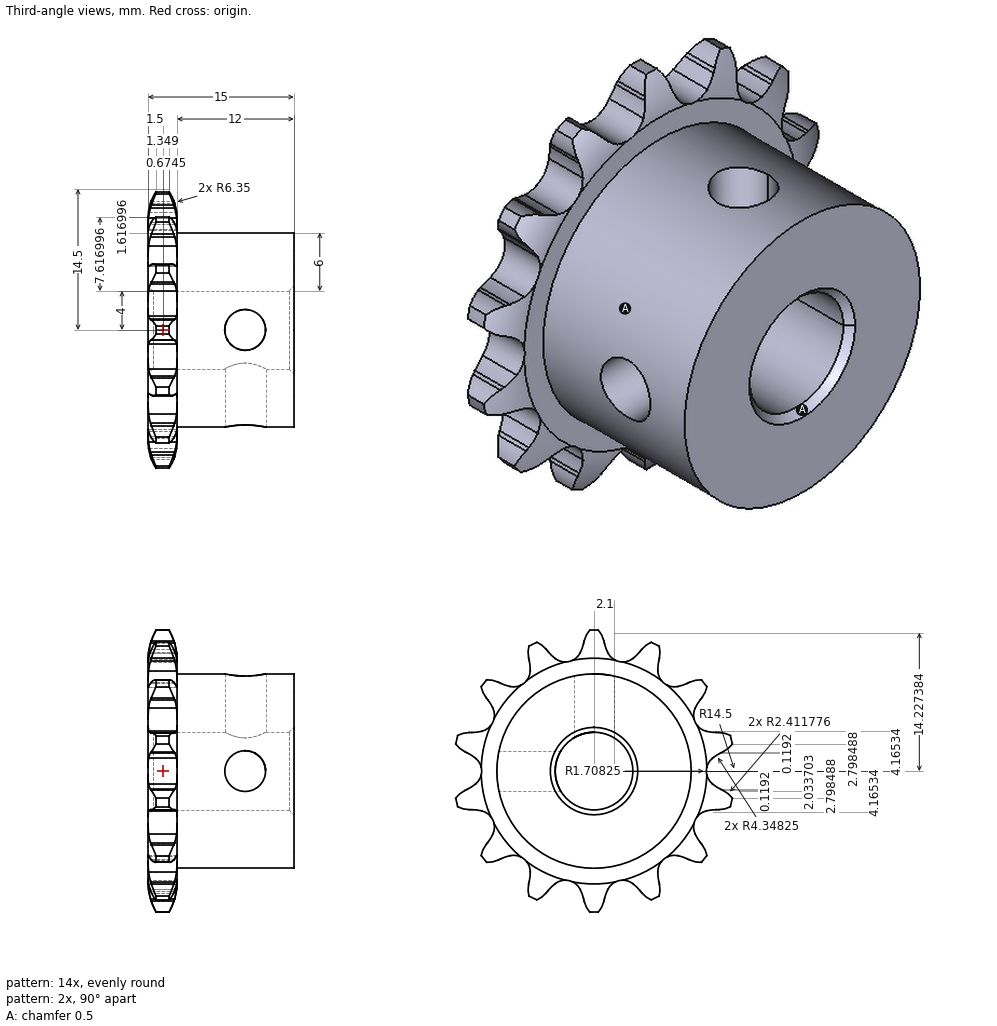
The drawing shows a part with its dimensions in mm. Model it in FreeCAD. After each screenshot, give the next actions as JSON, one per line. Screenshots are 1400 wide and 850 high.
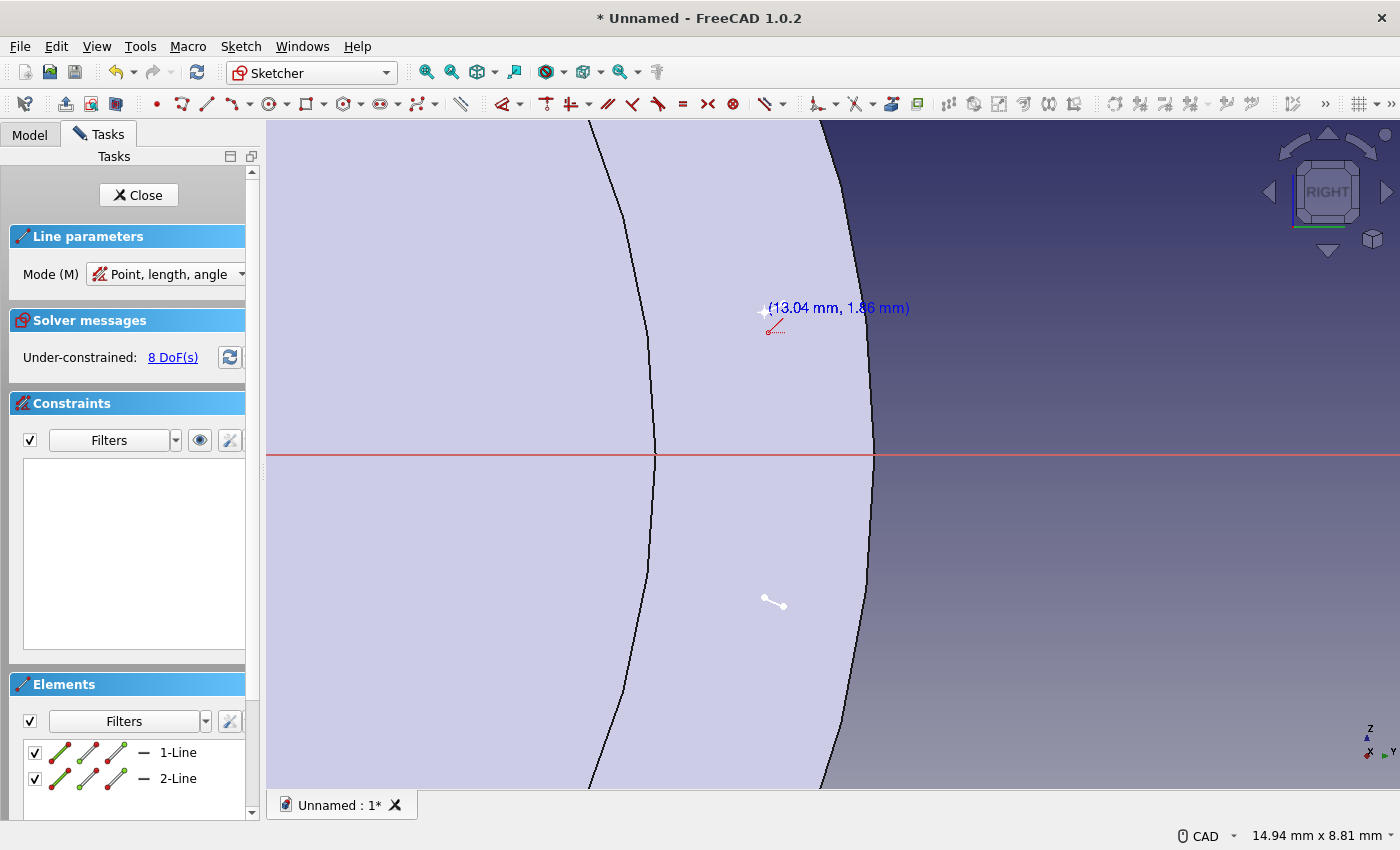
{"action": "left_click", "coordinate": [232, 104]}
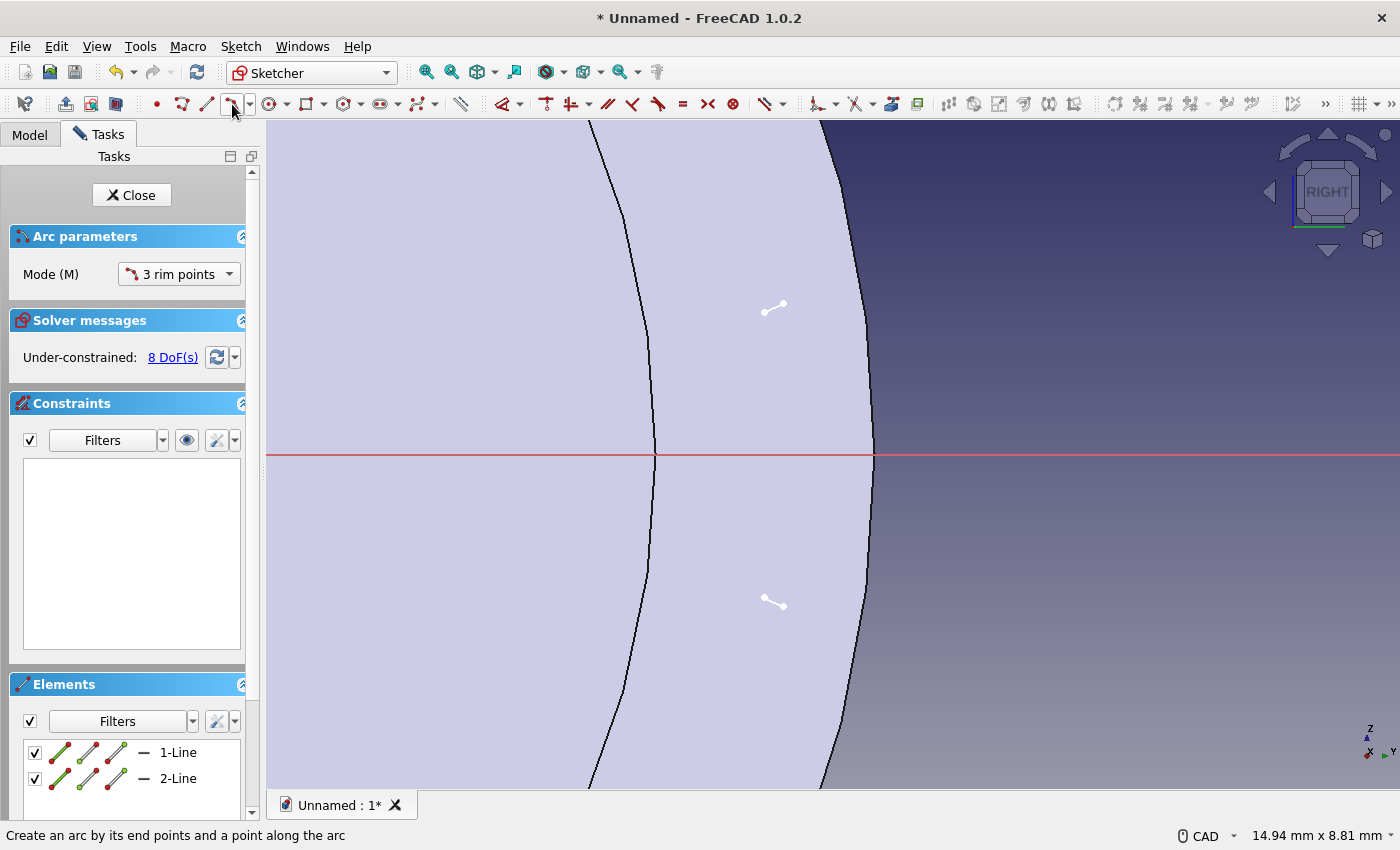
{"action": "scroll", "coordinate": [783, 606], "scroll_direction": "up", "scroll_amount": 3}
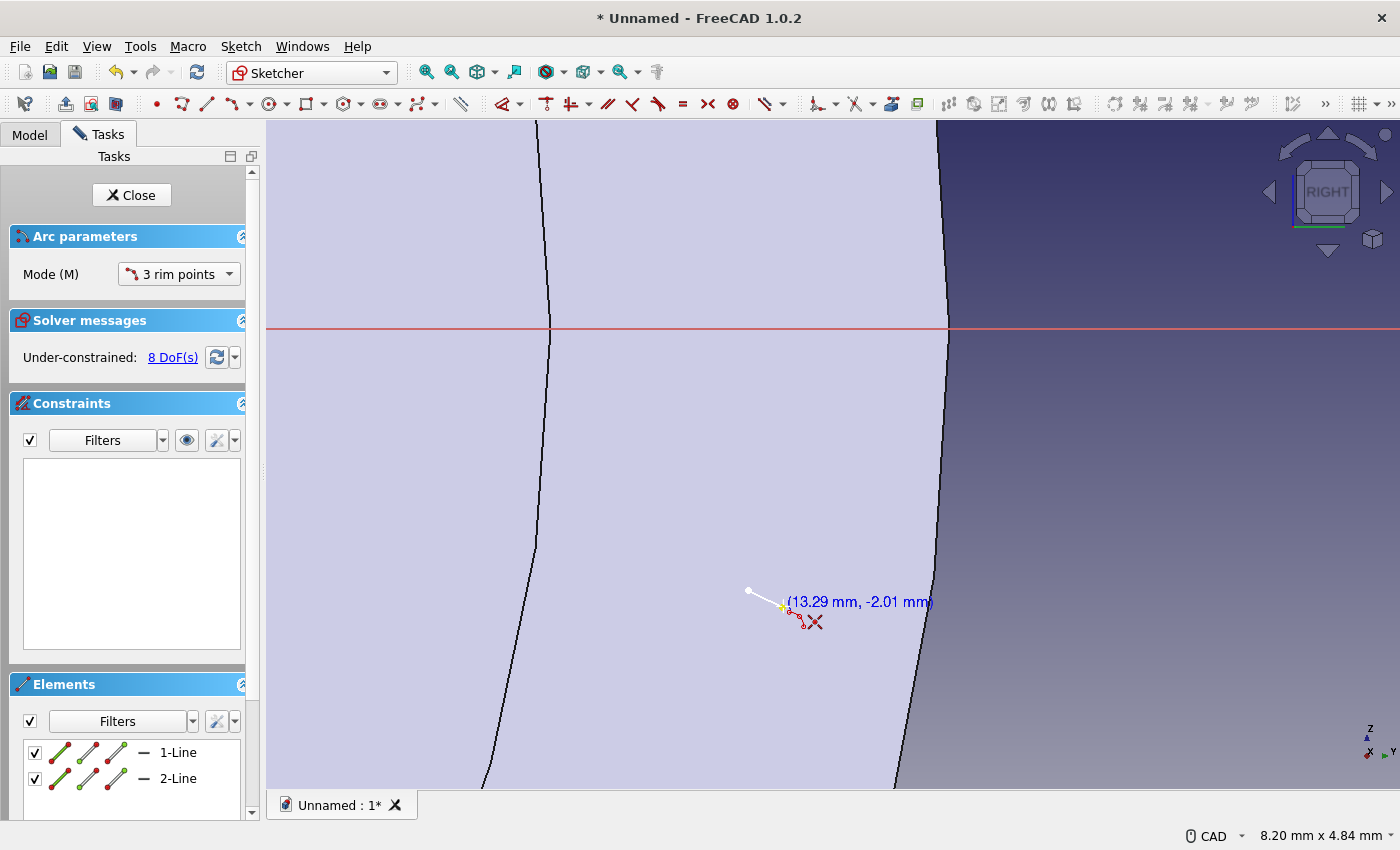
{"action": "left_click", "coordinate": [783, 607]}
{"action": "left_click", "coordinate": [912, 717]}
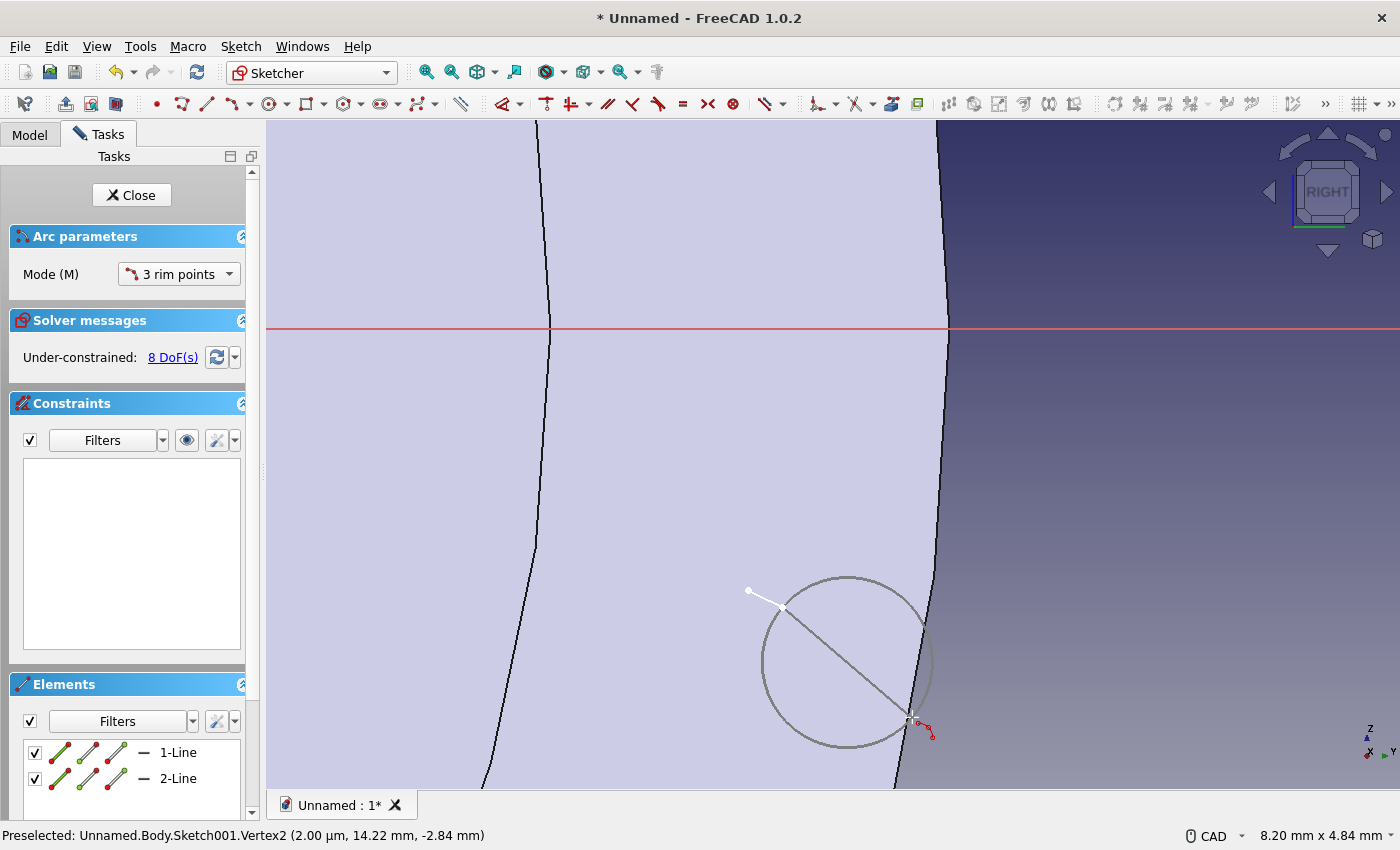
{"action": "scroll", "coordinate": [854, 653], "scroll_direction": "up", "scroll_amount": 2}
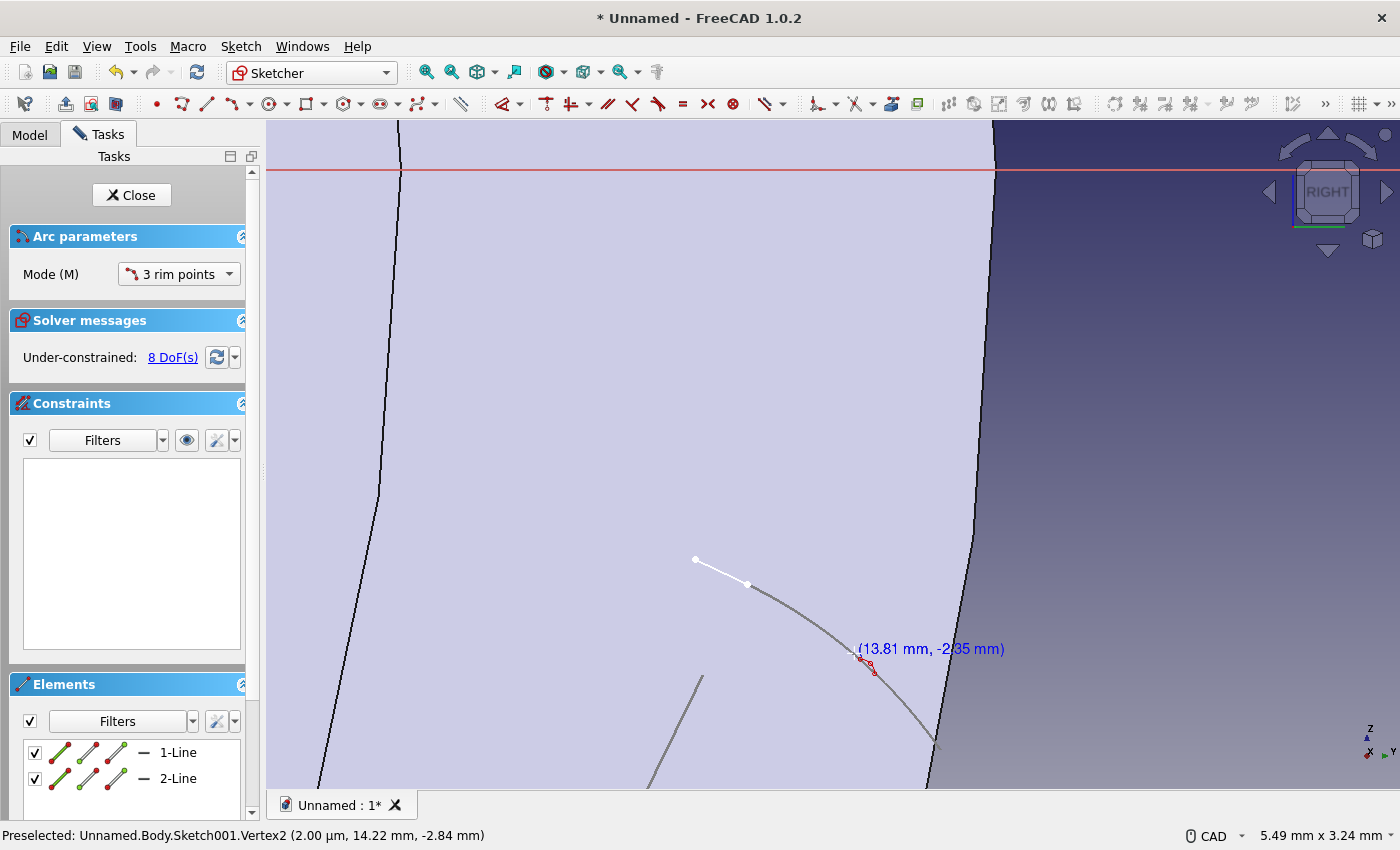
{"action": "left_click", "coordinate": [854, 652]}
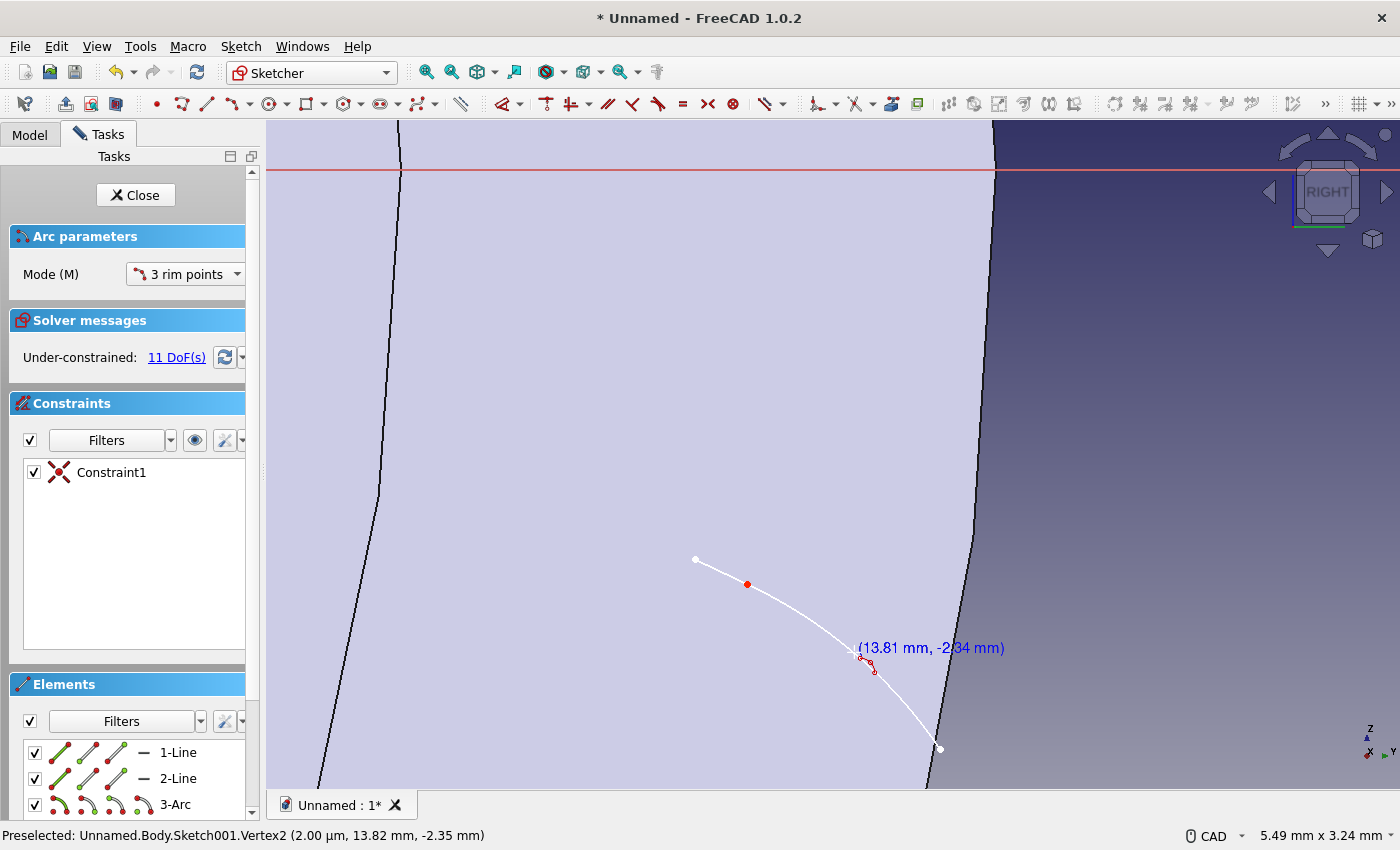
{"action": "left_click", "coordinate": [940, 750]}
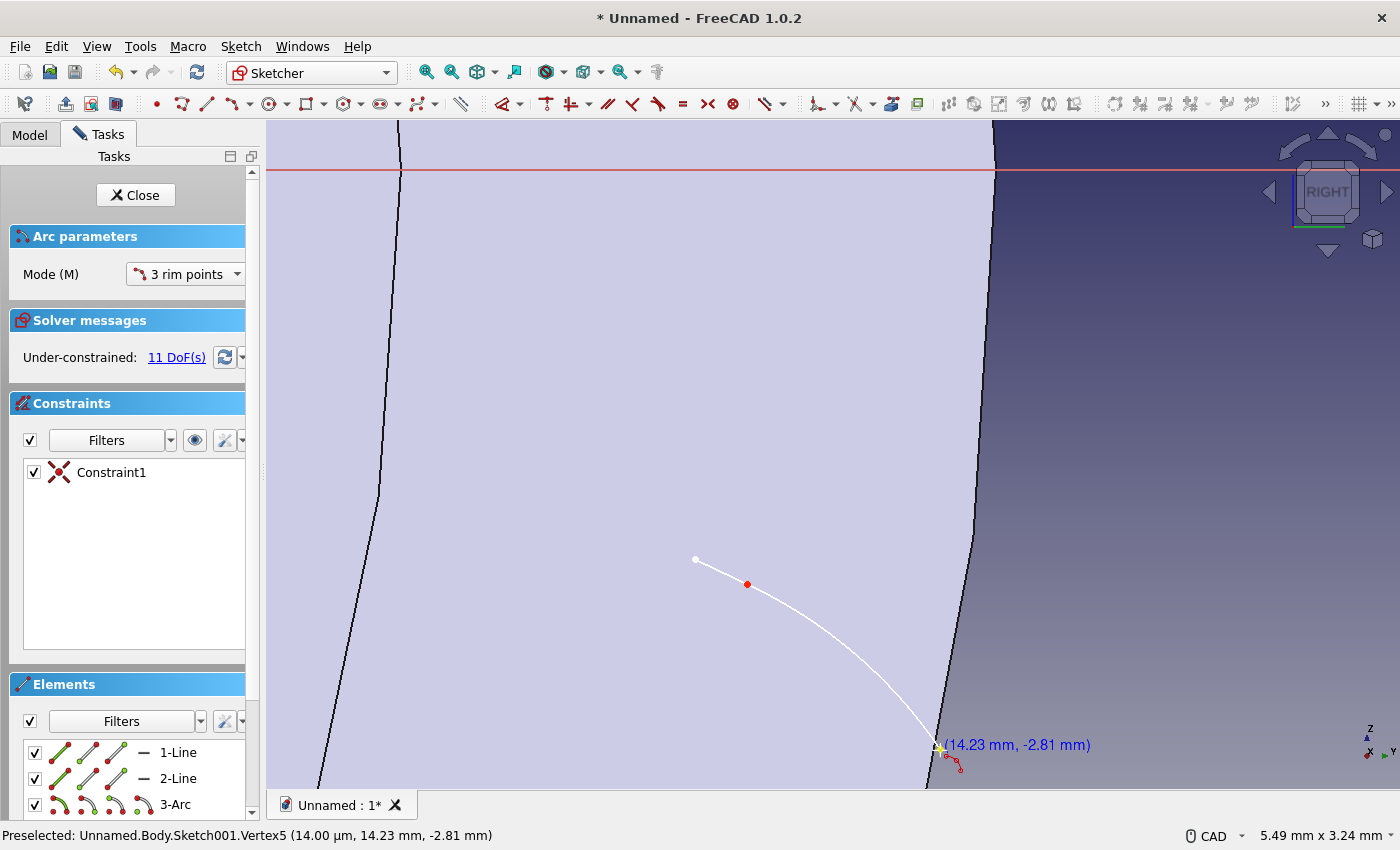
{"action": "scroll", "coordinate": [806, 620], "scroll_direction": "down", "scroll_amount": 5}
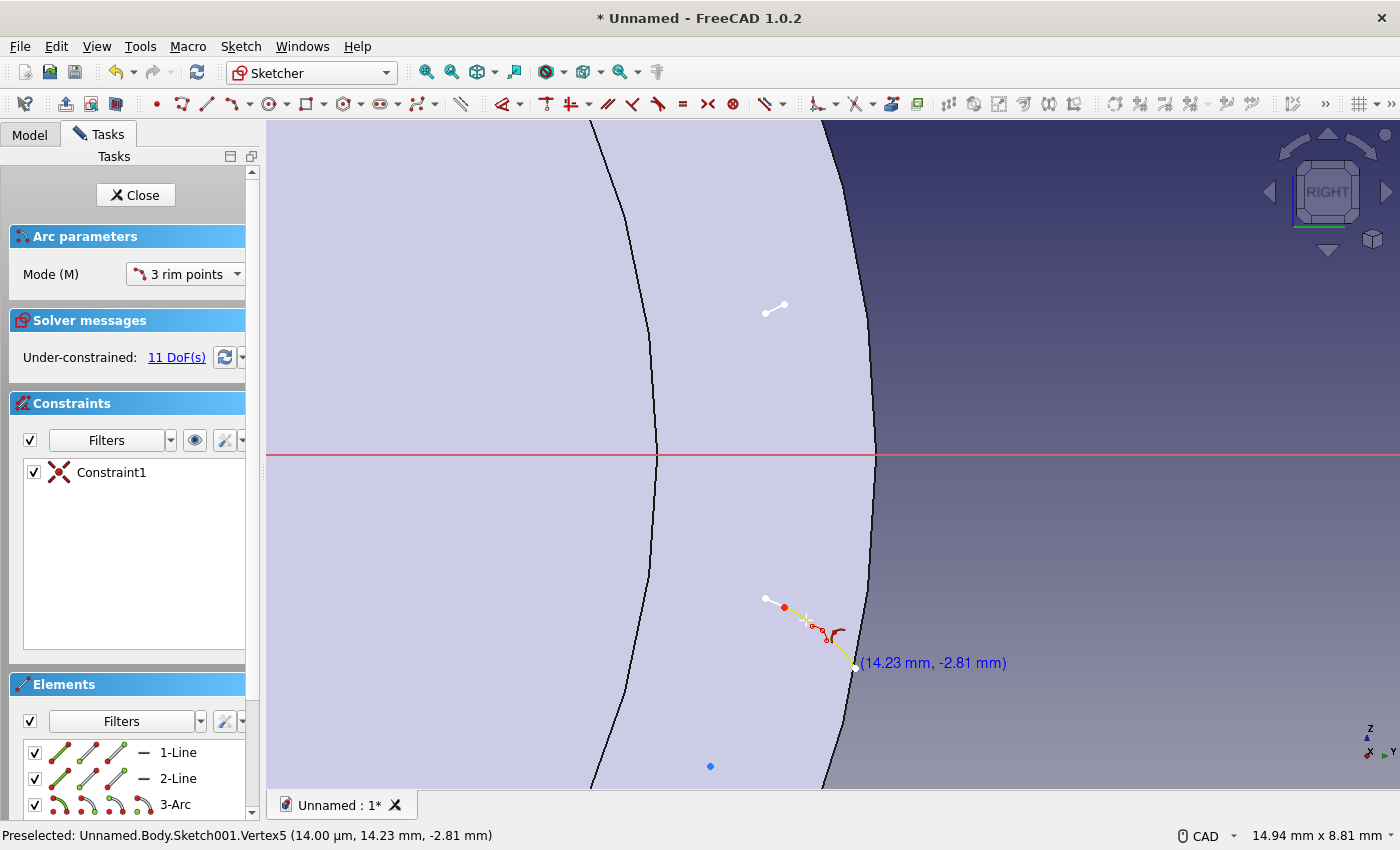
{"action": "left_click", "coordinate": [856, 242]}
{"action": "left_click", "coordinate": [875, 498]}